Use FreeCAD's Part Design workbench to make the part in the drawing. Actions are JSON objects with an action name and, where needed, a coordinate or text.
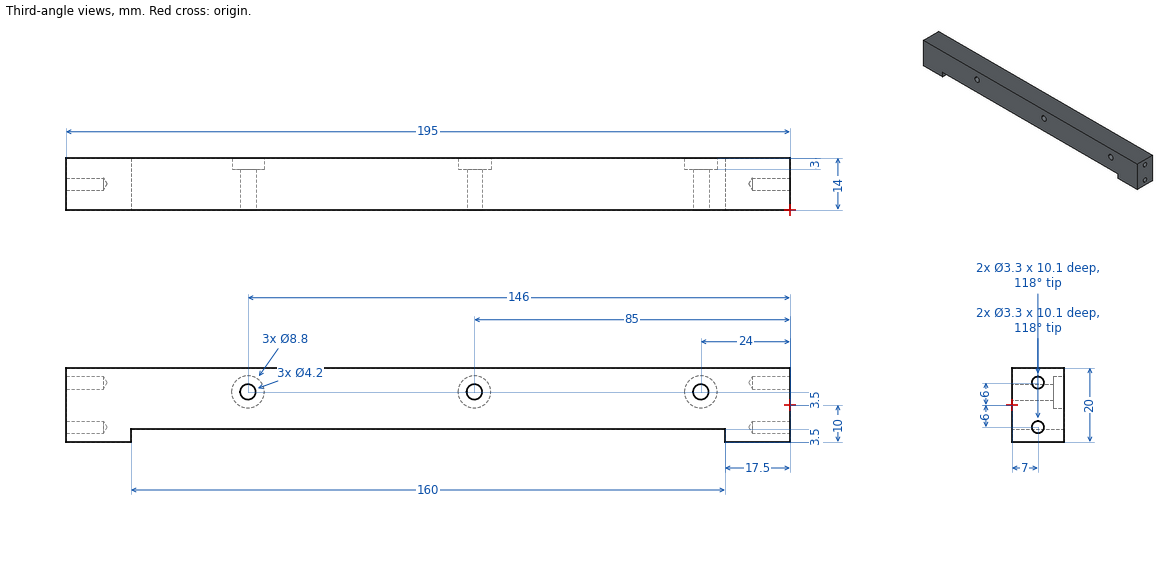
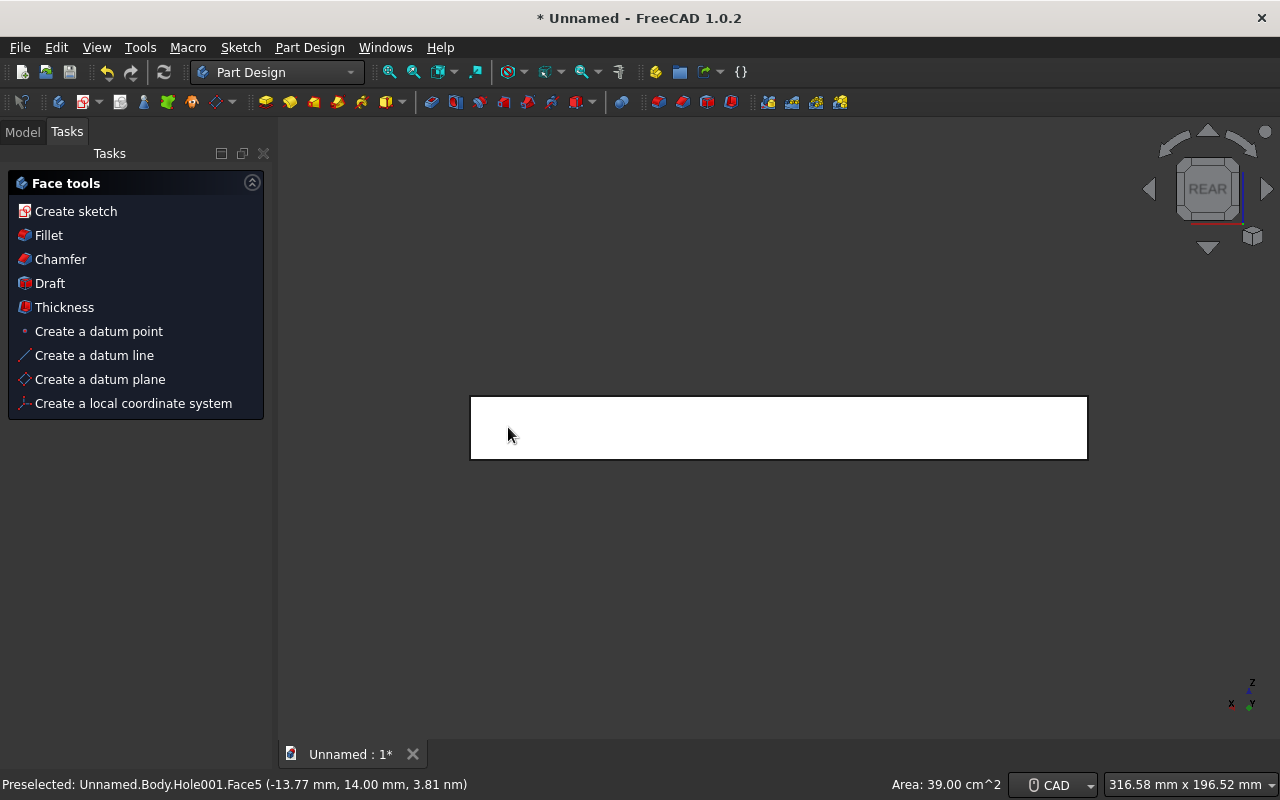
{"action": "left_click", "coordinate": [84, 102]}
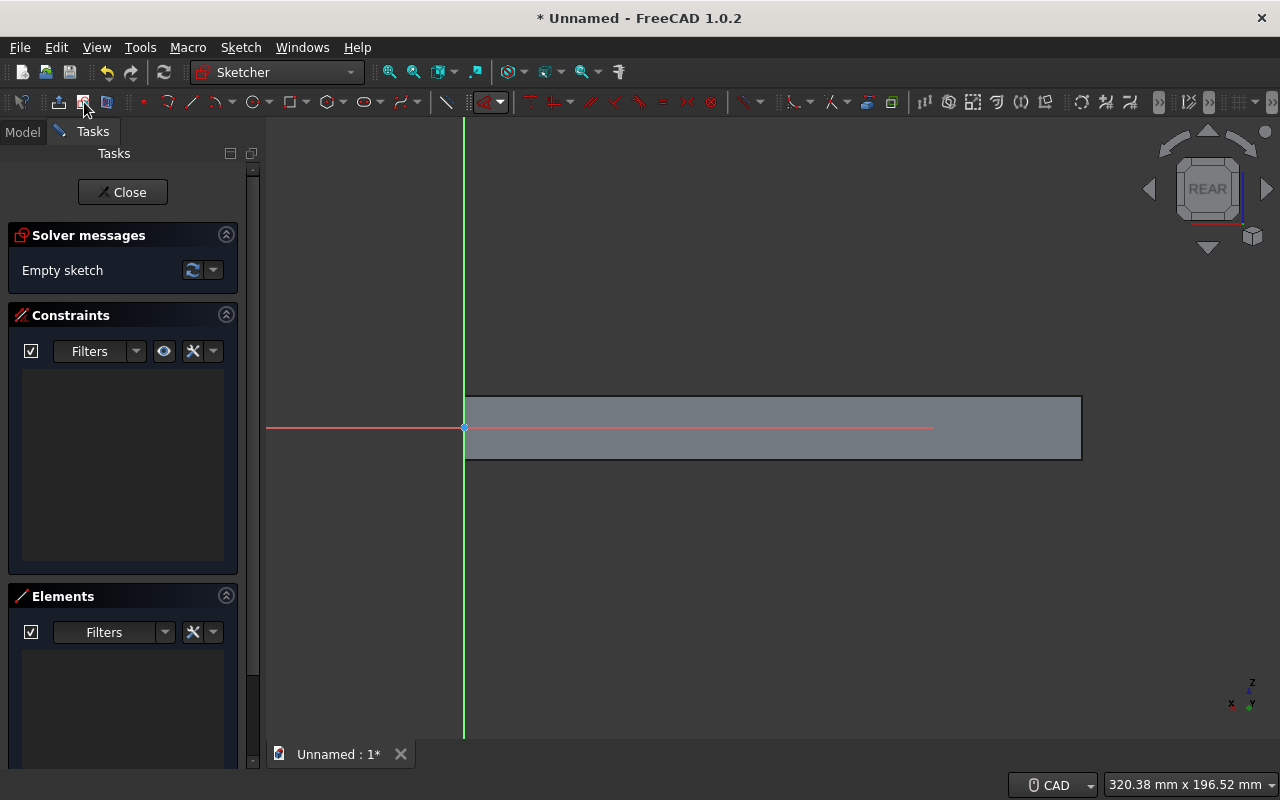
{"action": "key", "text": "g c"}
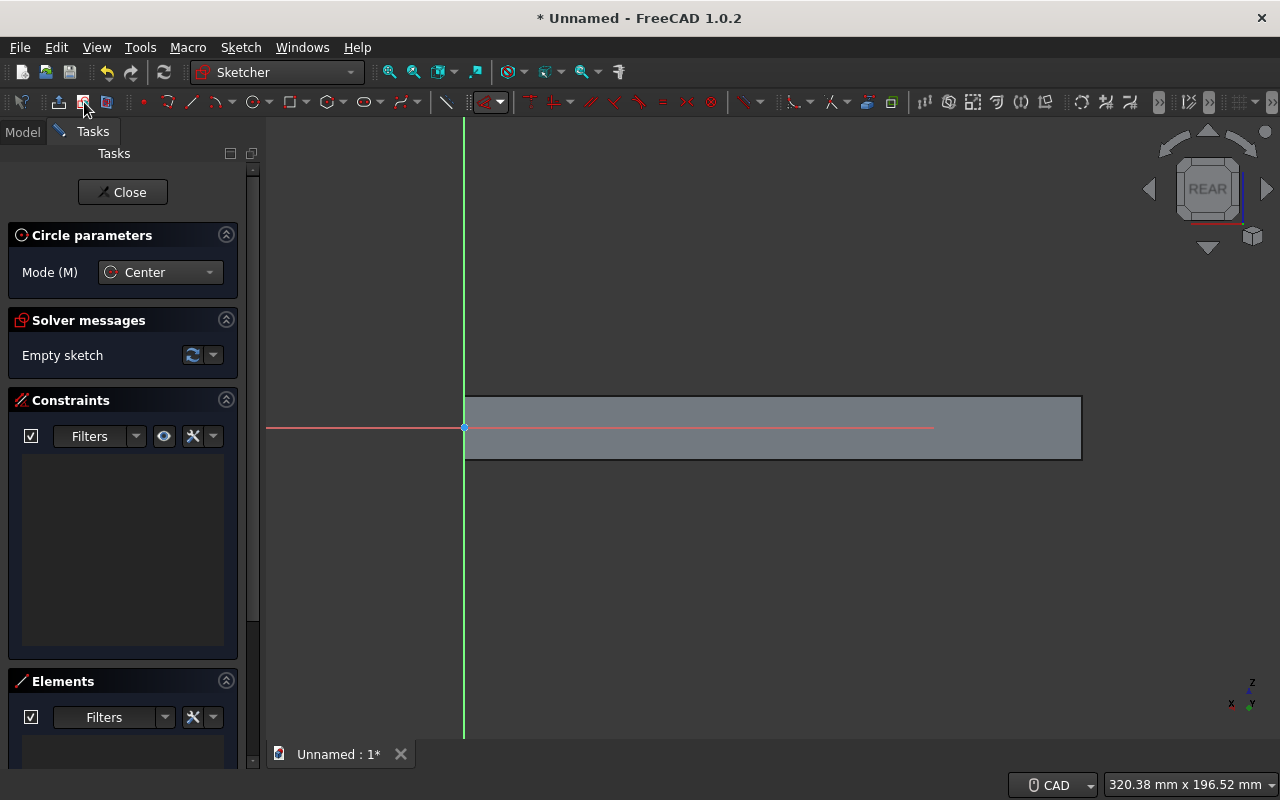
{"action": "scroll", "coordinate": [927, 417], "scroll_direction": "up", "scroll_amount": 7}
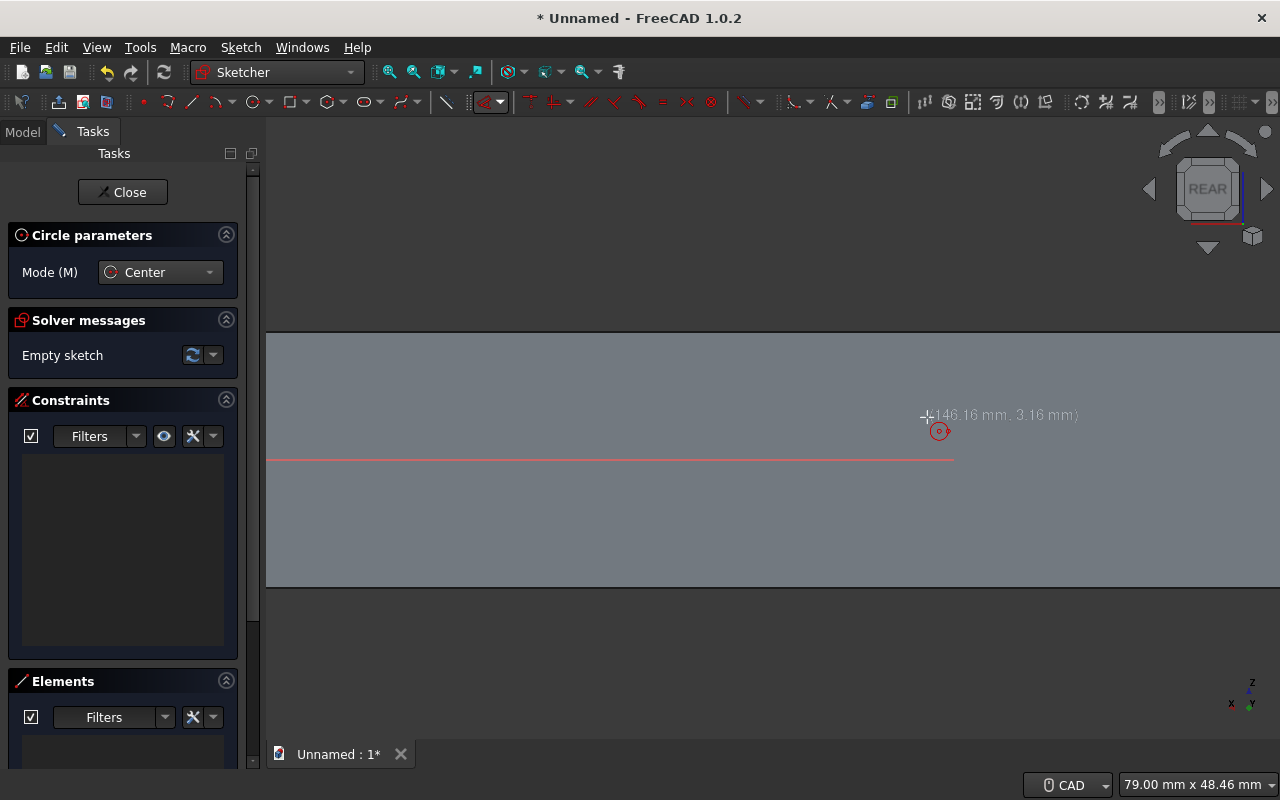
{"action": "left_click", "coordinate": [923, 415]}
{"action": "left_click", "coordinate": [942, 396]}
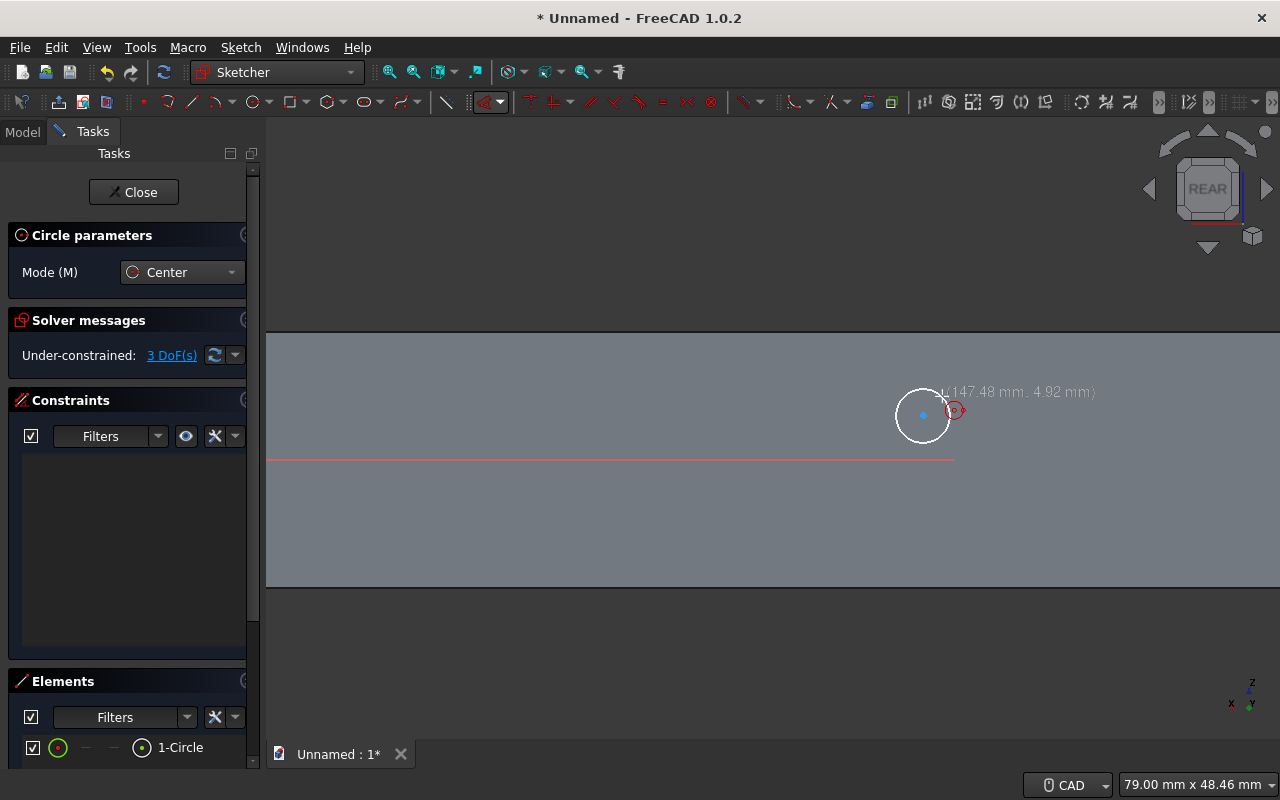
{"action": "scroll", "coordinate": [1008, 430], "scroll_direction": "down", "scroll_amount": 6}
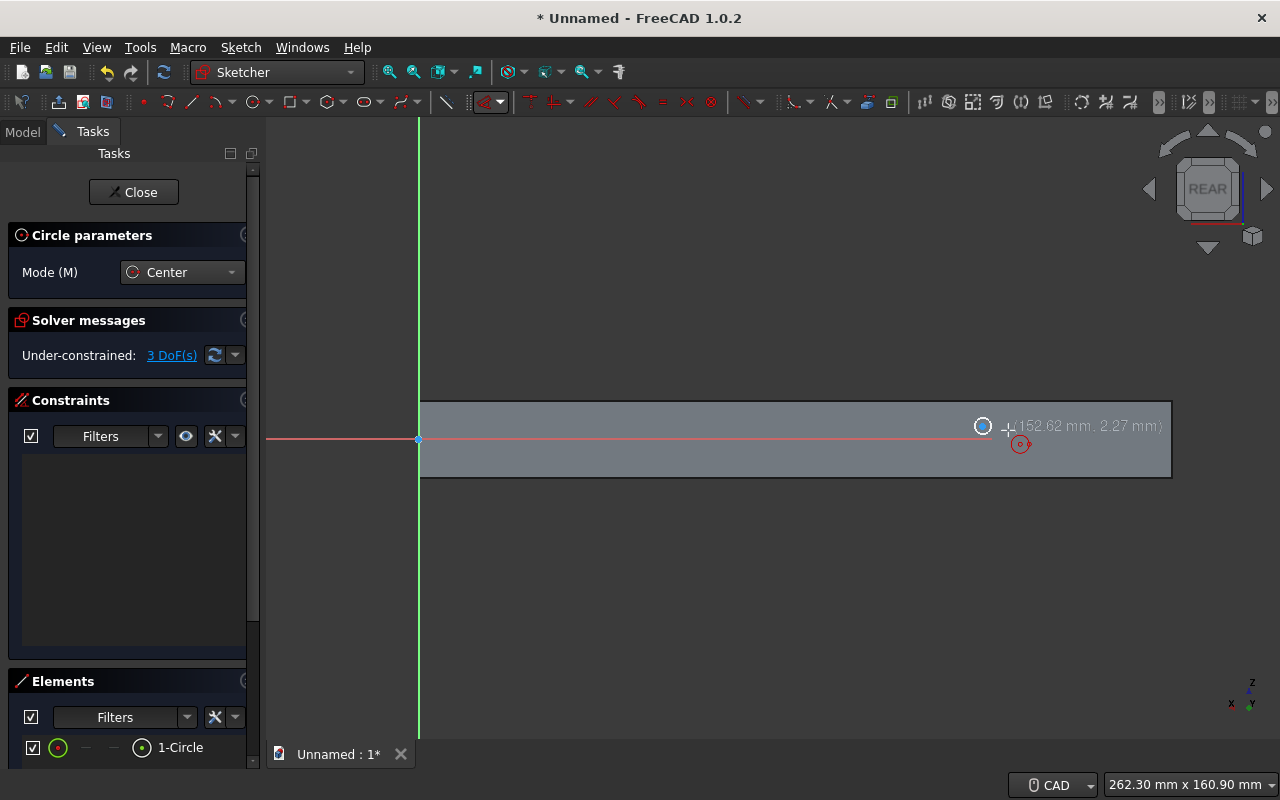
{"action": "scroll", "coordinate": [747, 426], "scroll_direction": "up", "scroll_amount": 6}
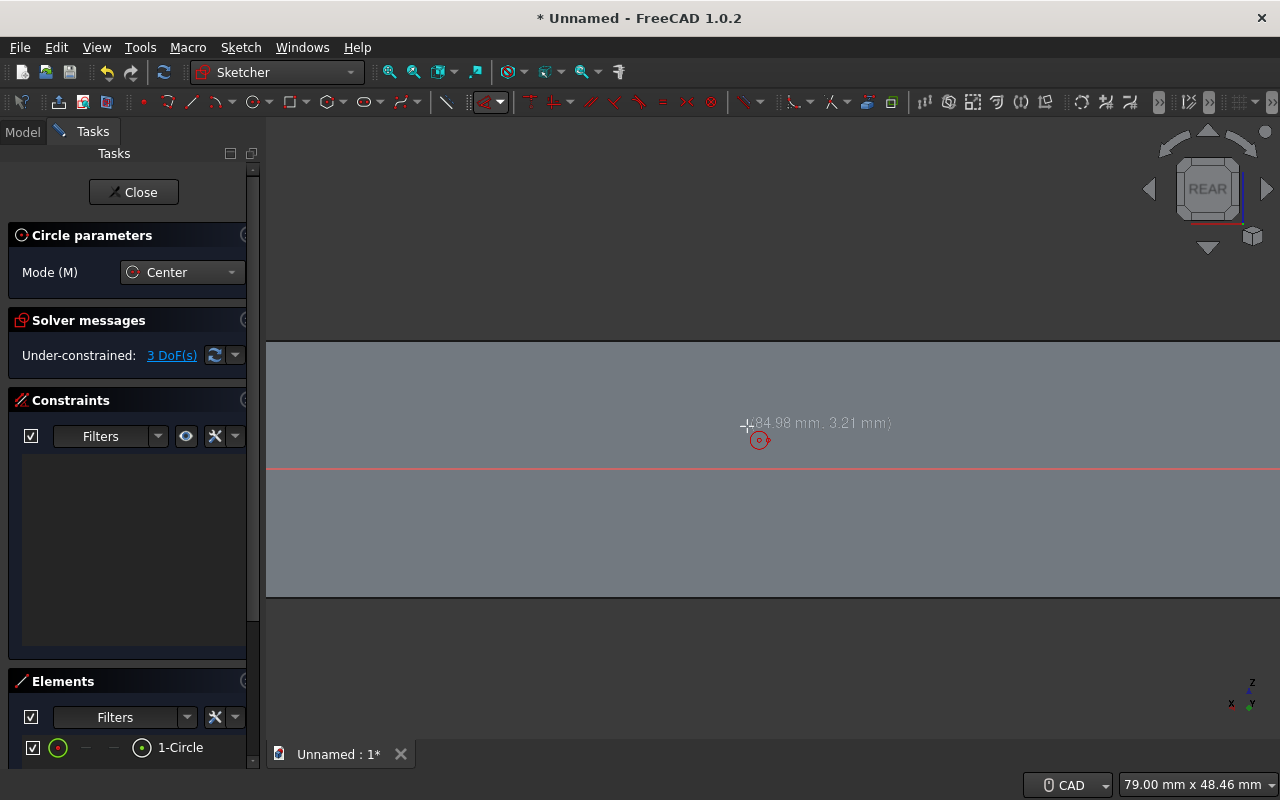
{"action": "left_click", "coordinate": [746, 425]}
{"action": "left_click", "coordinate": [765, 405]}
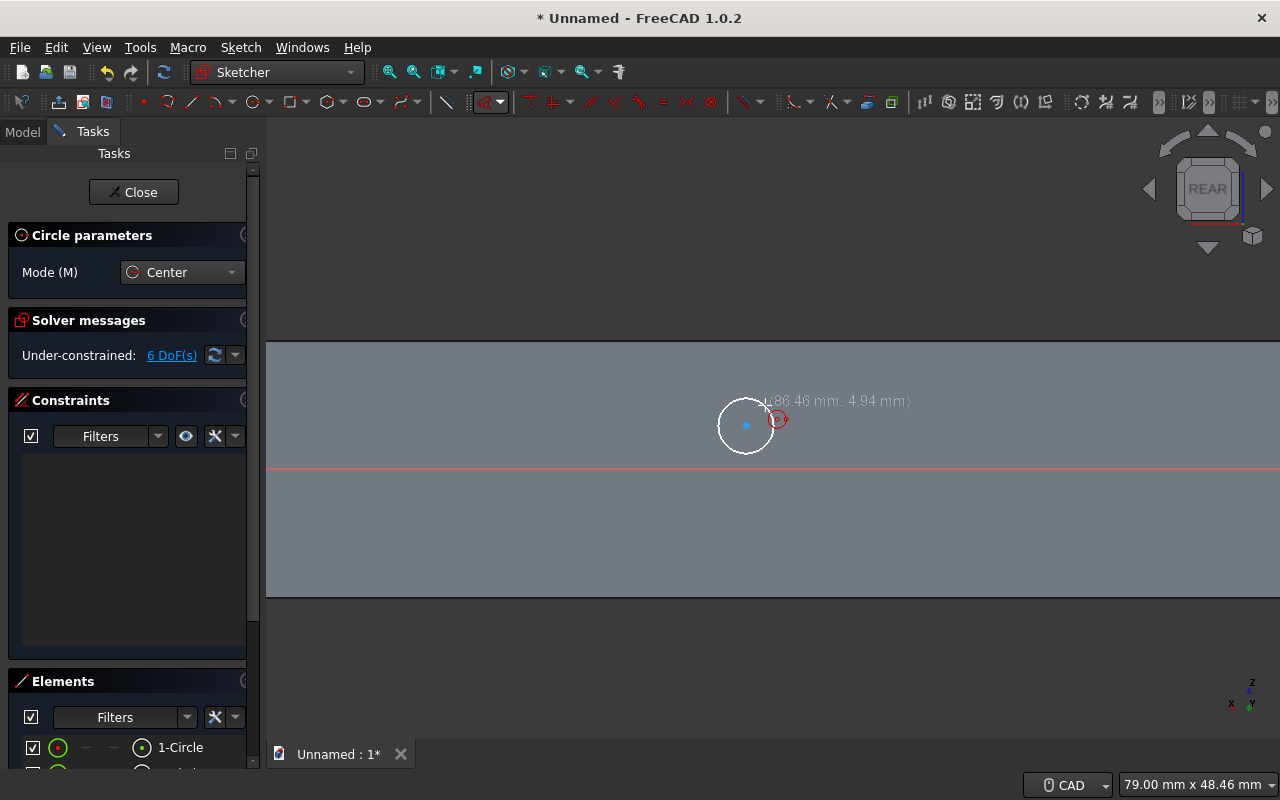
{"action": "scroll", "coordinate": [747, 426], "scroll_direction": "down", "scroll_amount": 6}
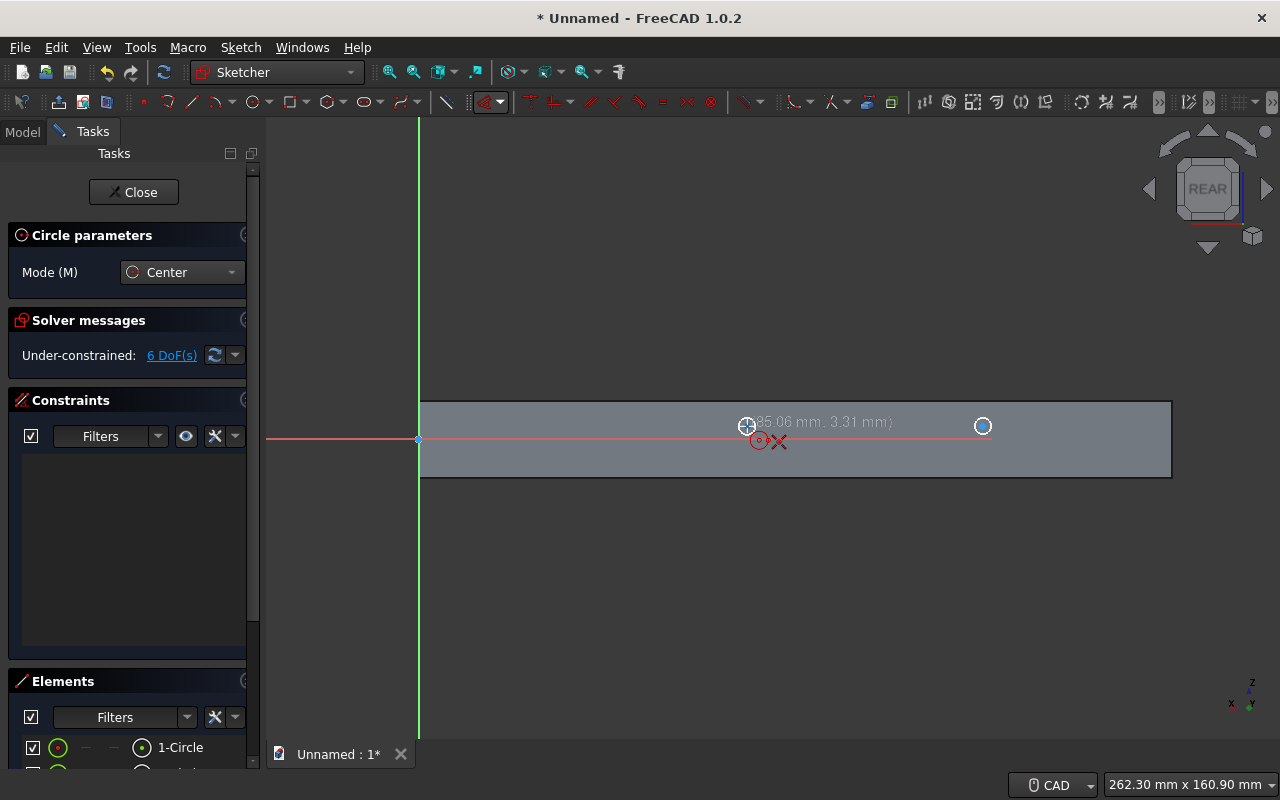
{"action": "scroll", "coordinate": [511, 426], "scroll_direction": "up", "scroll_amount": 6}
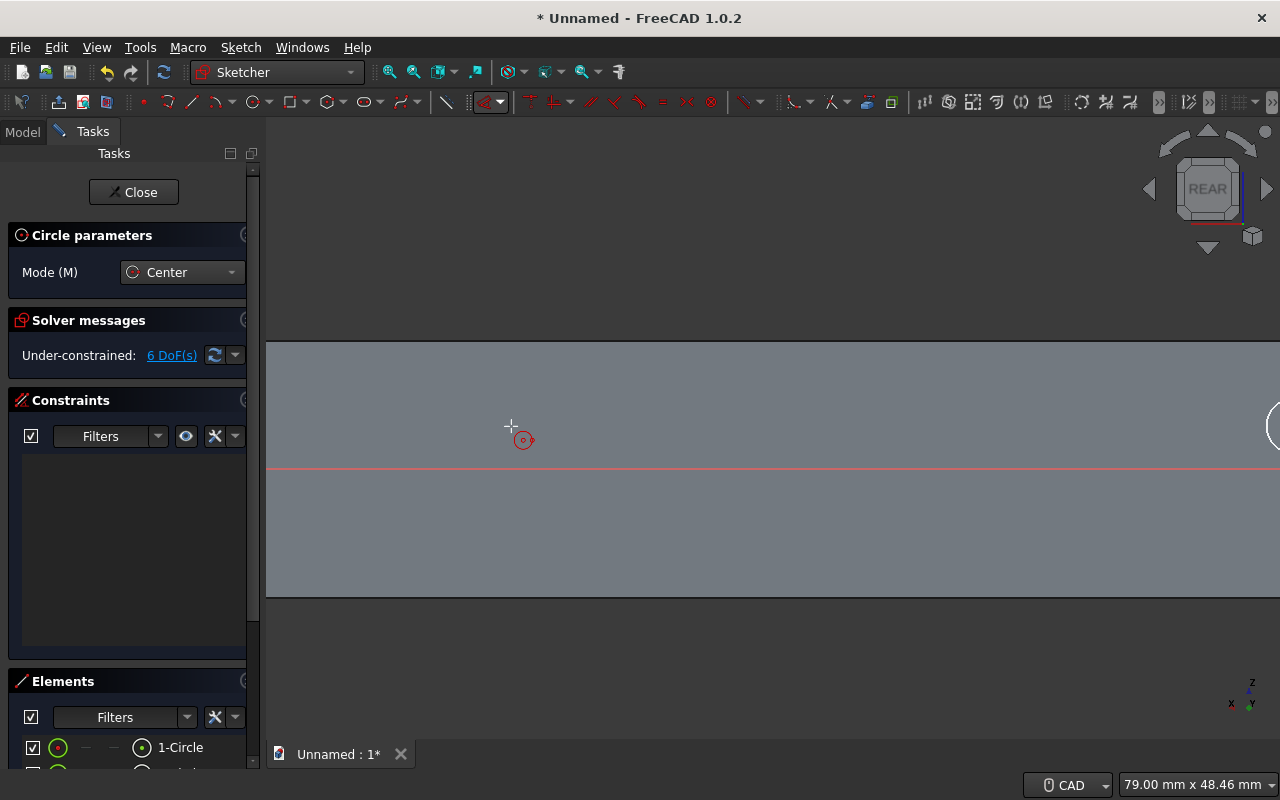
{"action": "left_click", "coordinate": [511, 425]}
{"action": "left_click", "coordinate": [530, 405]}
{"action": "key", "text": "Escape"}